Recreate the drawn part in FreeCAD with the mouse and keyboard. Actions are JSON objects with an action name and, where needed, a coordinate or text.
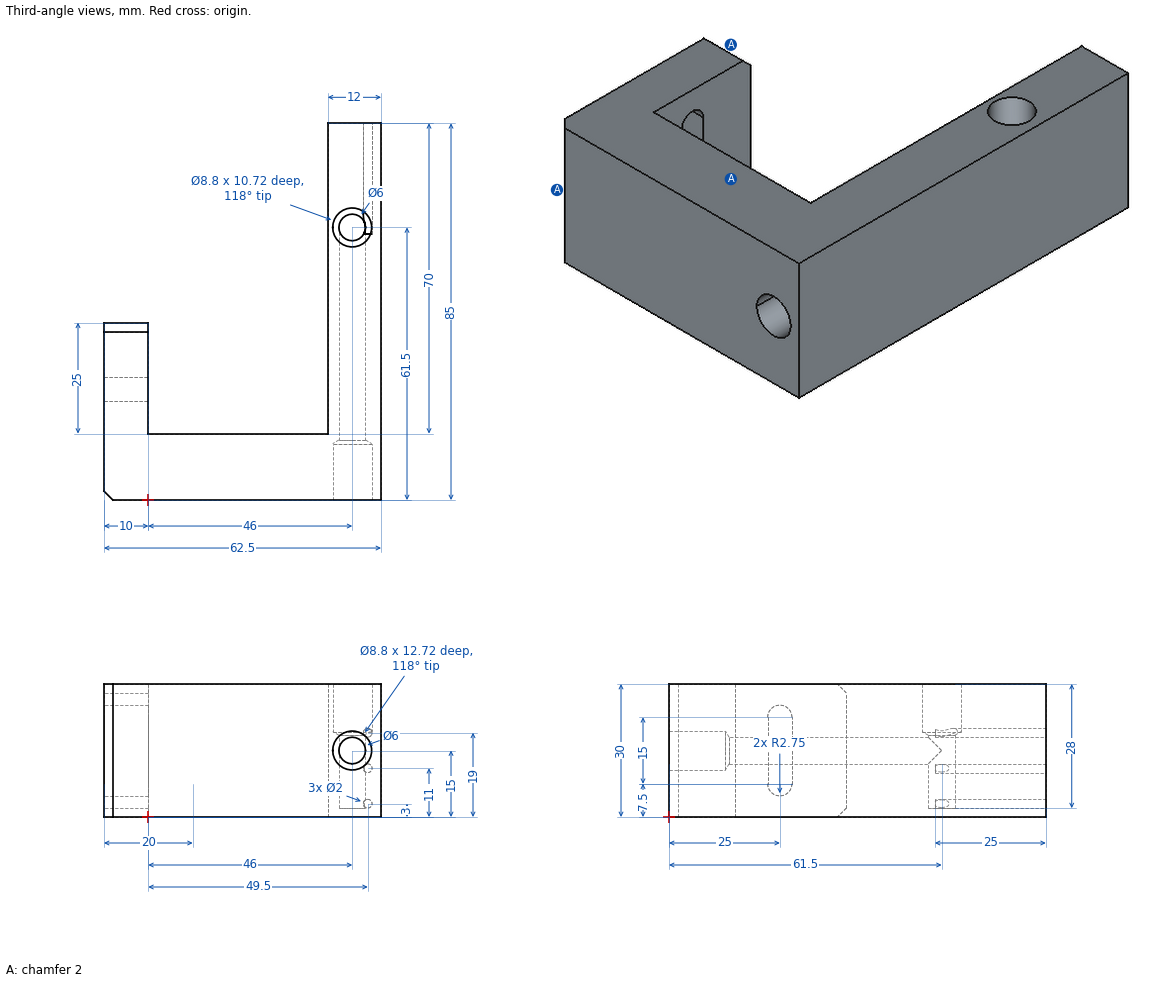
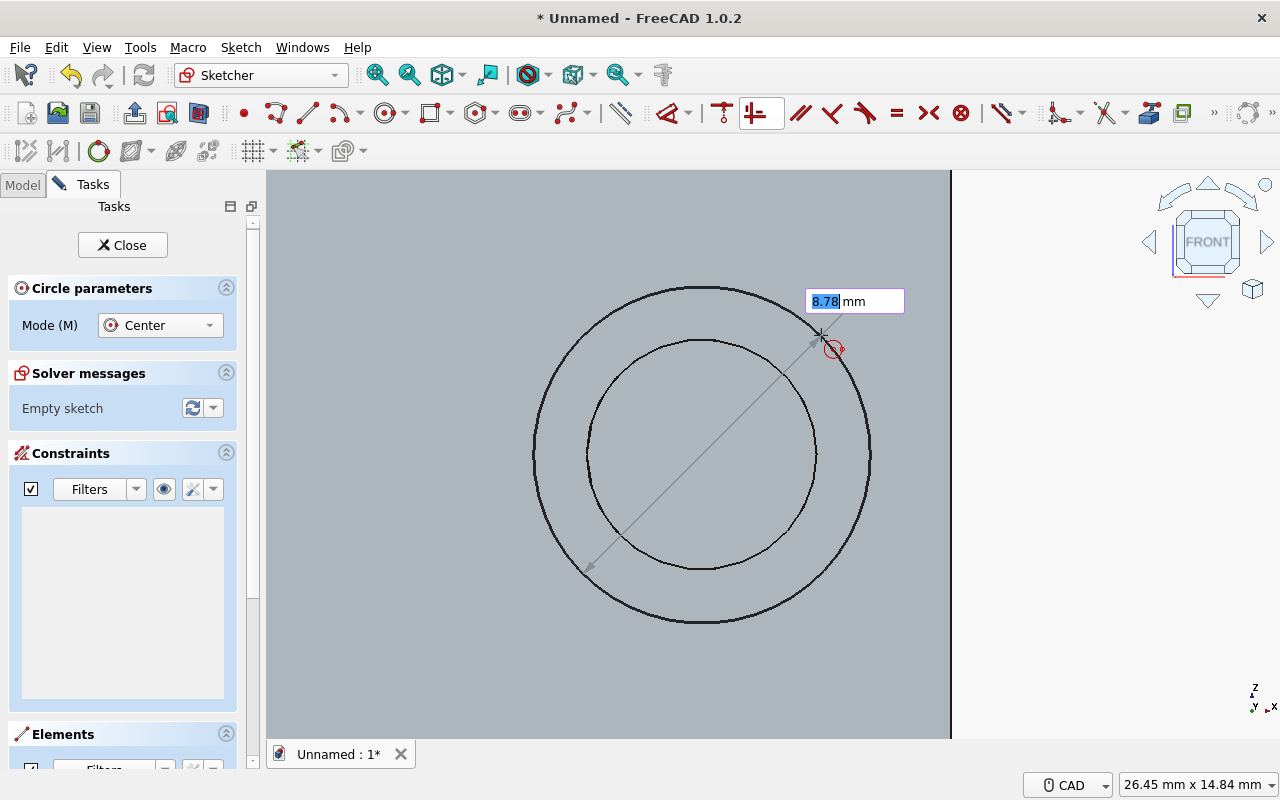
{"action": "type", "text": "8.8"}
{"action": "key", "text": "Return"}
{"action": "key", "text": "Escape"}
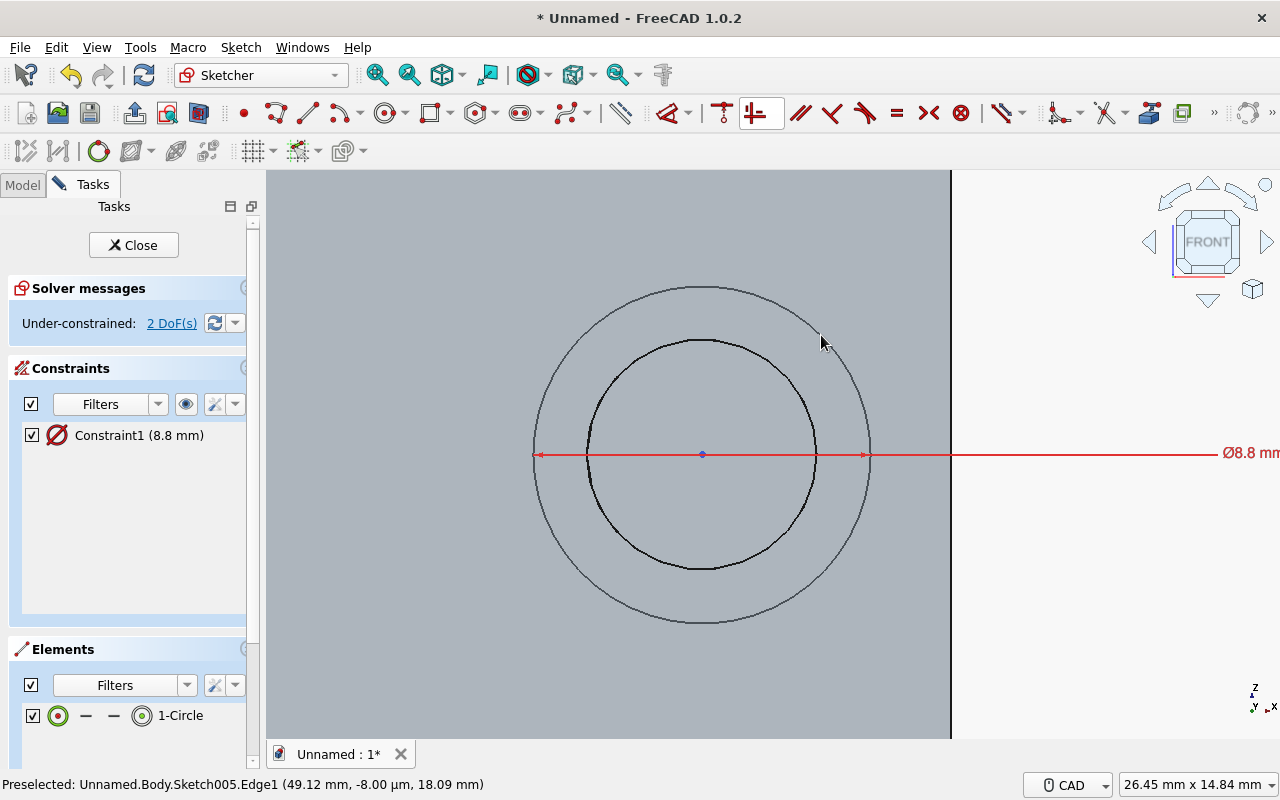
{"action": "key", "text": "d"}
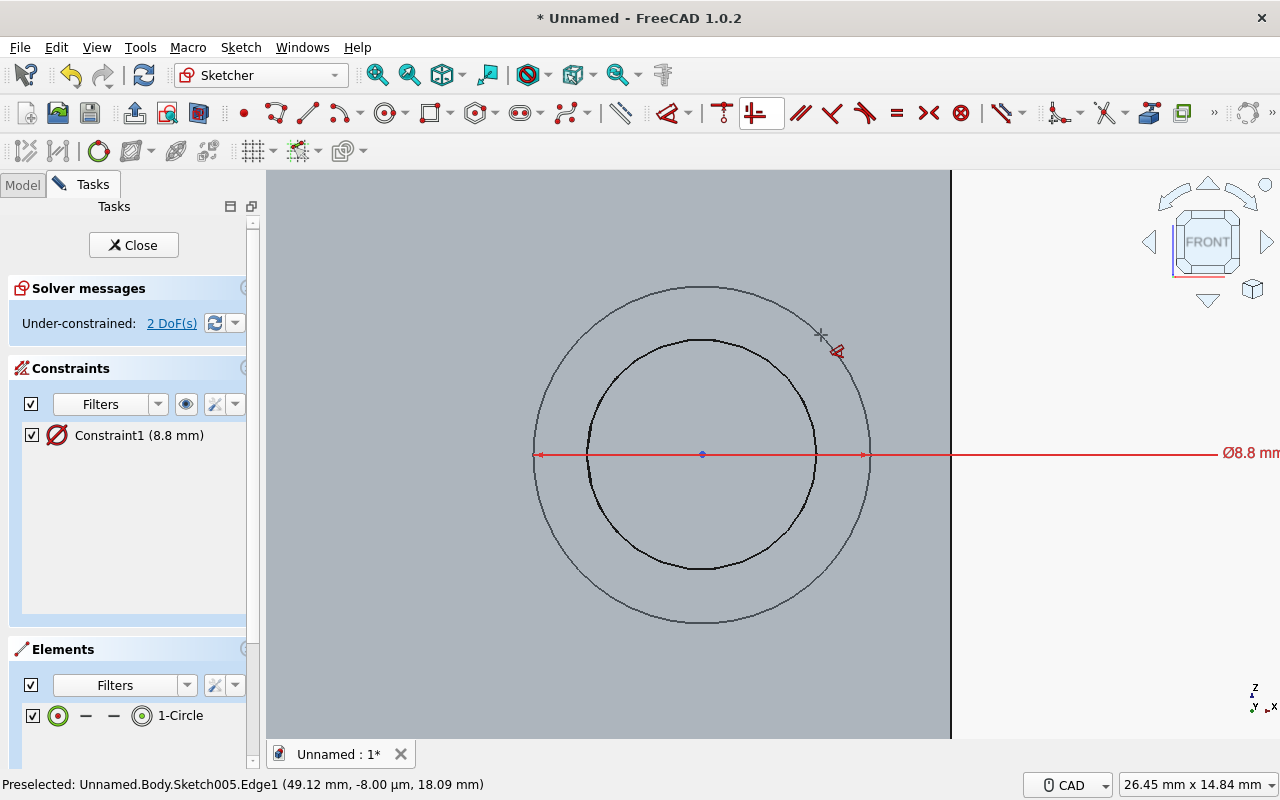
{"action": "left_click", "coordinate": [702, 455]}
{"action": "left_click", "coordinate": [498, 421]}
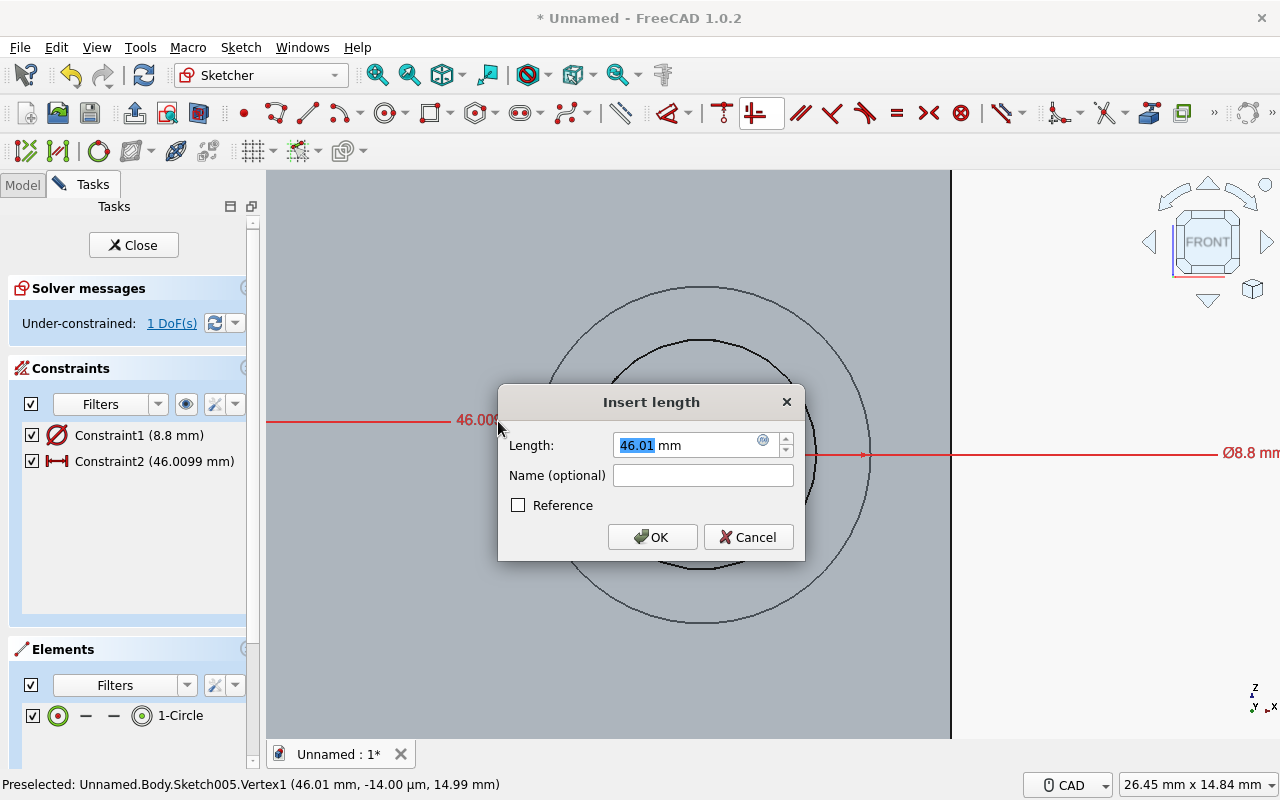
{"action": "type", "text": "46"}
{"action": "key", "text": "Return"}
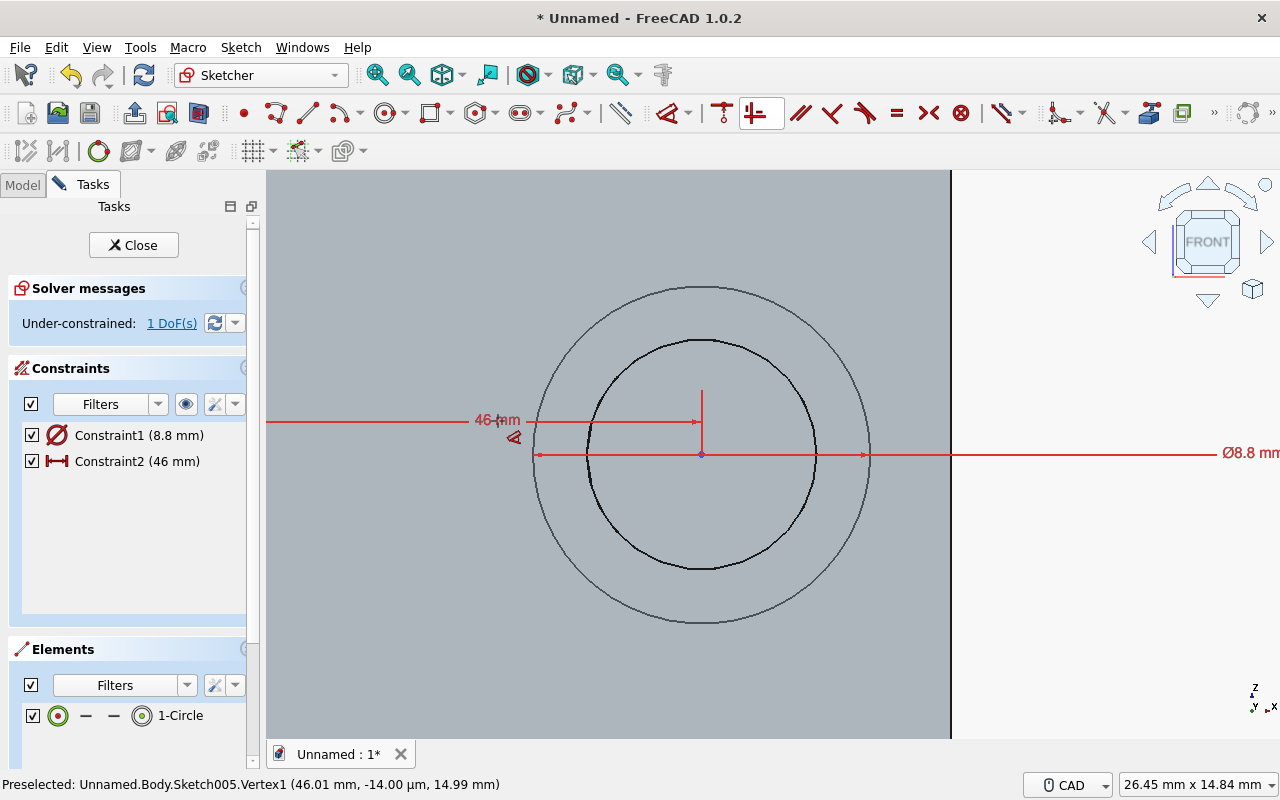
{"action": "left_click", "coordinate": [702, 455]}
{"action": "left_click", "coordinate": [736, 583]}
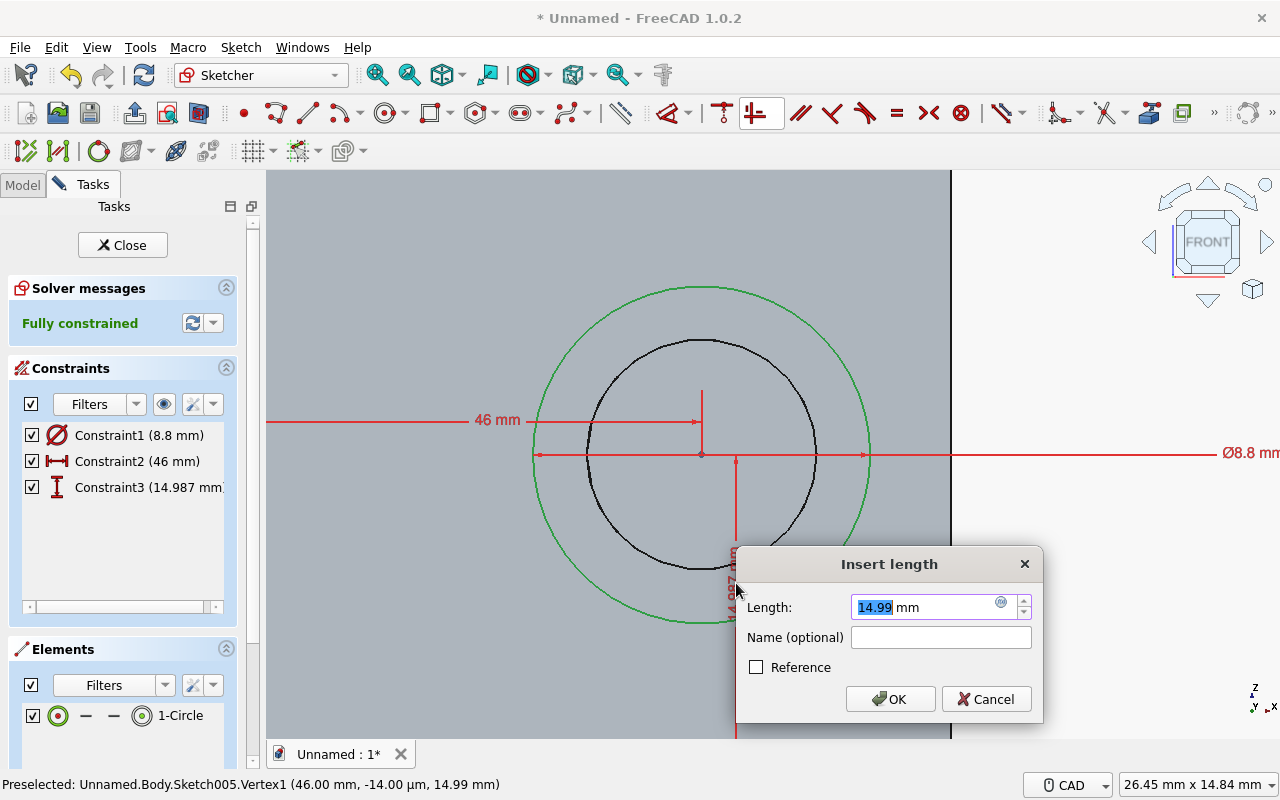
{"action": "type", "text": "15"}
{"action": "key", "text": "Return"}
{"action": "key", "text": "Escape"}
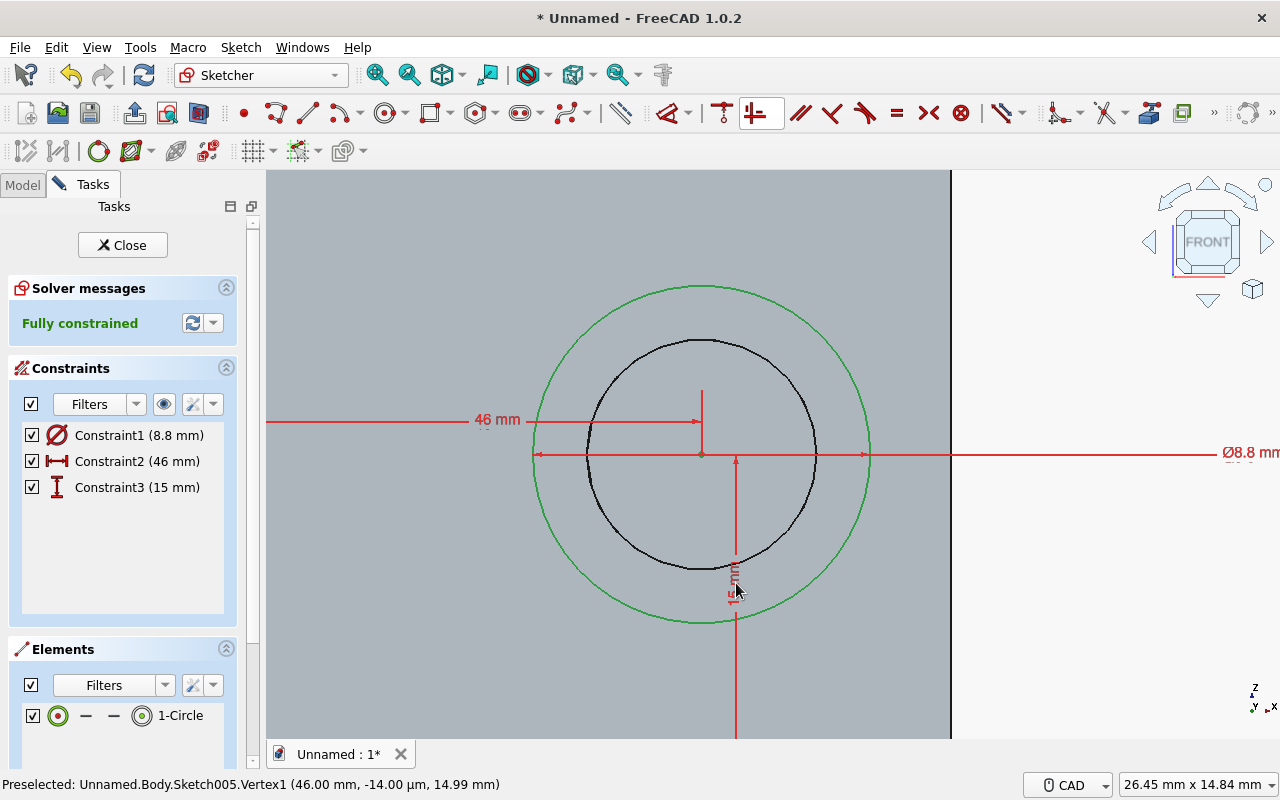
{"action": "left_click", "coordinate": [123, 245]}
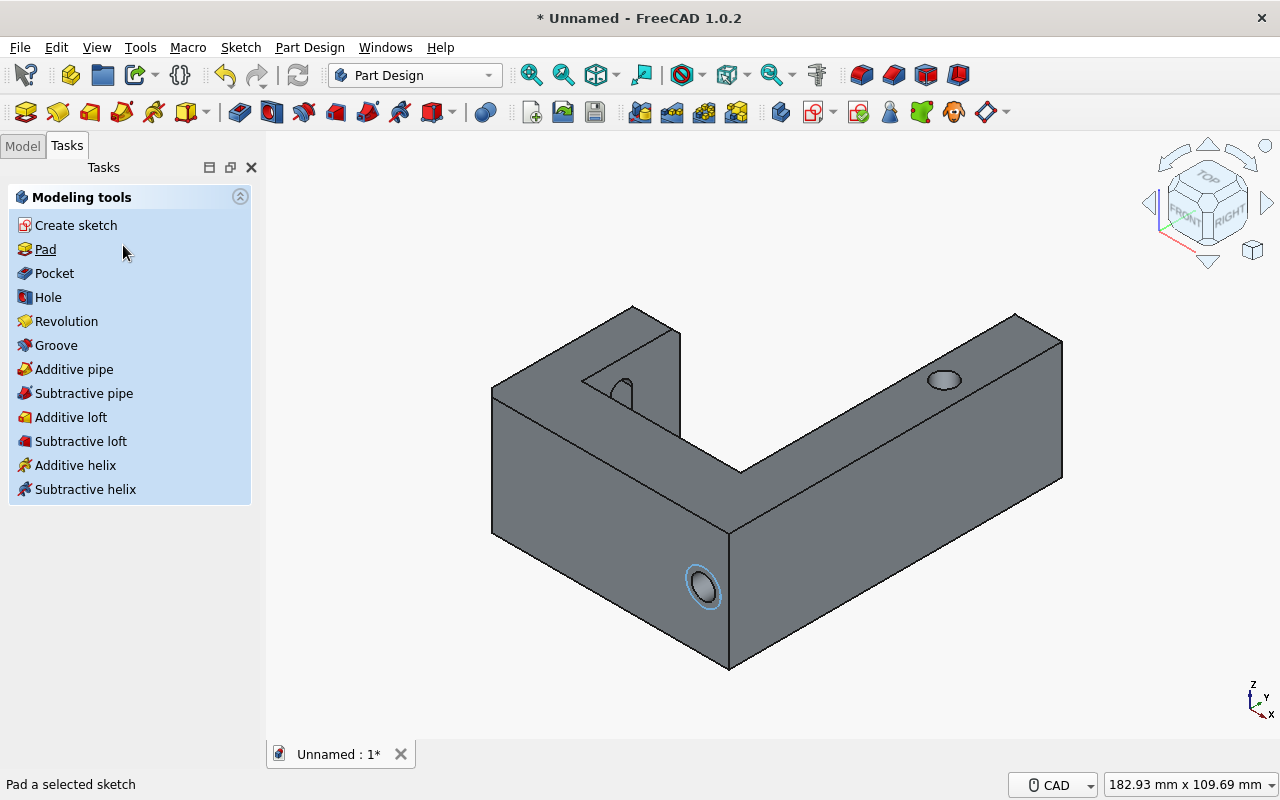
{"action": "left_click", "coordinate": [272, 112]}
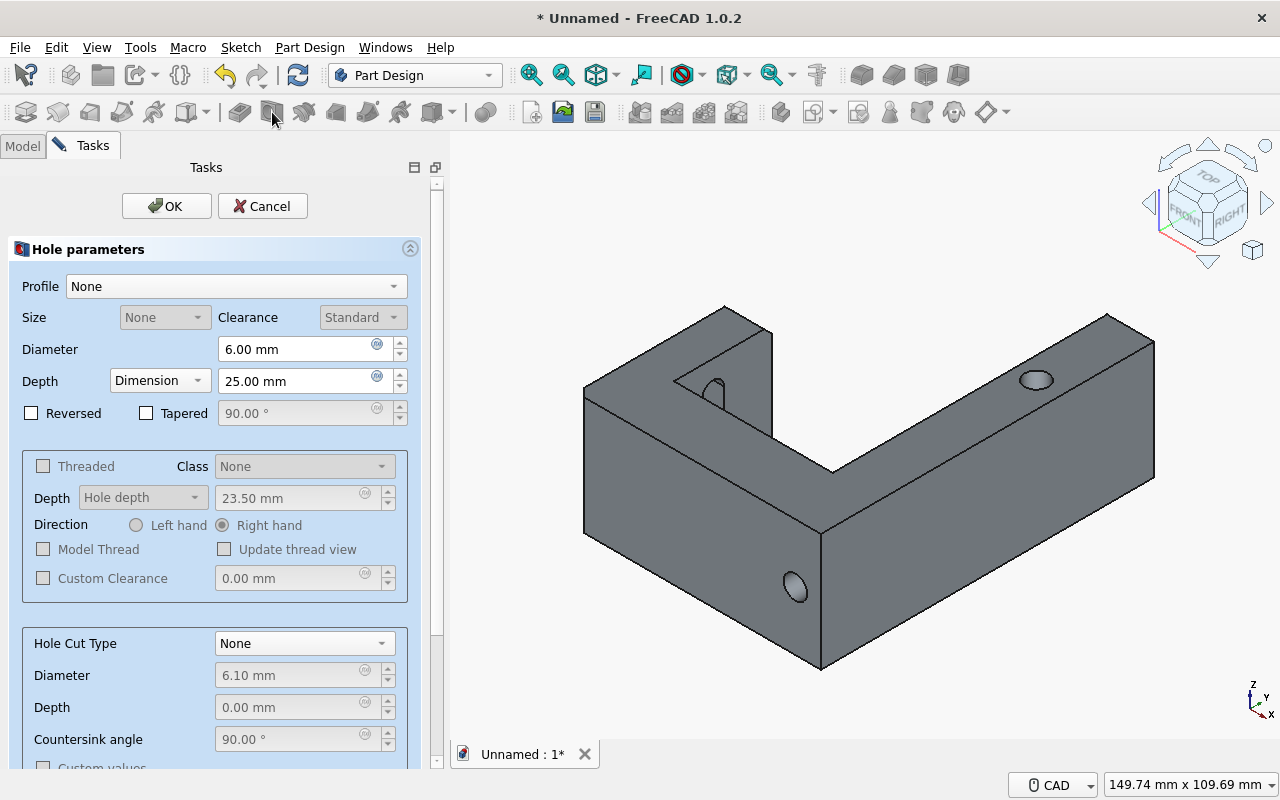
{"action": "triple_click", "coordinate": [305, 349]}